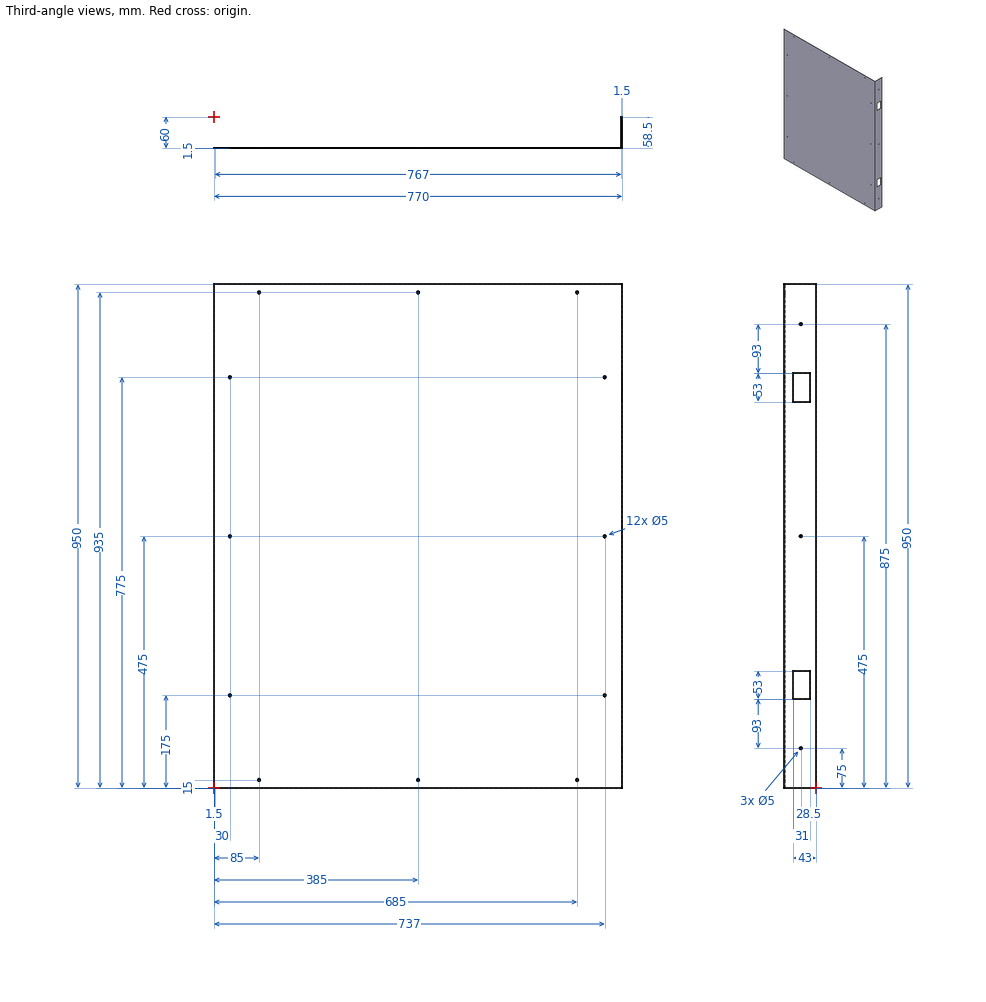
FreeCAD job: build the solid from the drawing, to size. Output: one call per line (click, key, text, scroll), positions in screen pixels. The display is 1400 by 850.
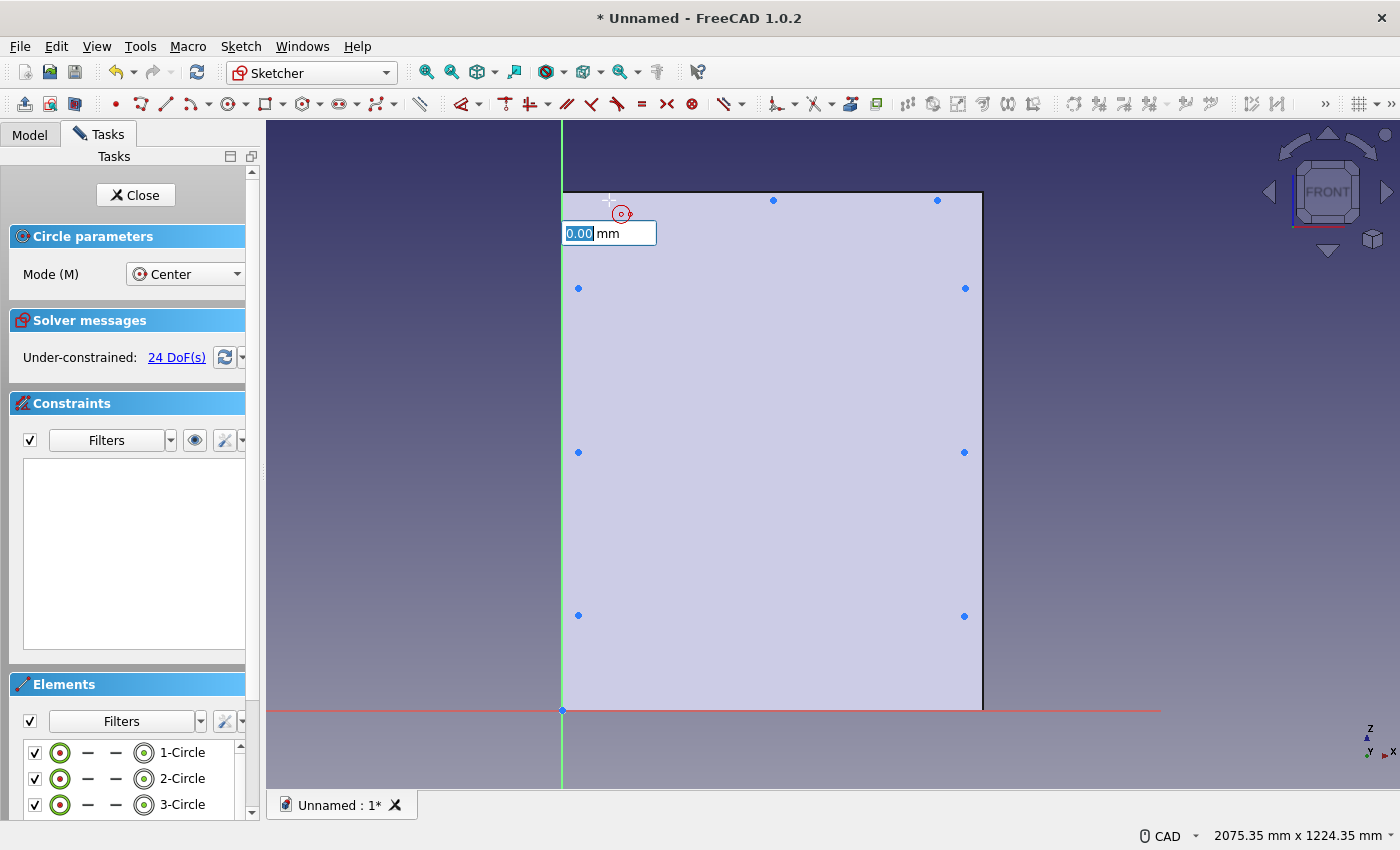
scroll(610, 199, up, 13)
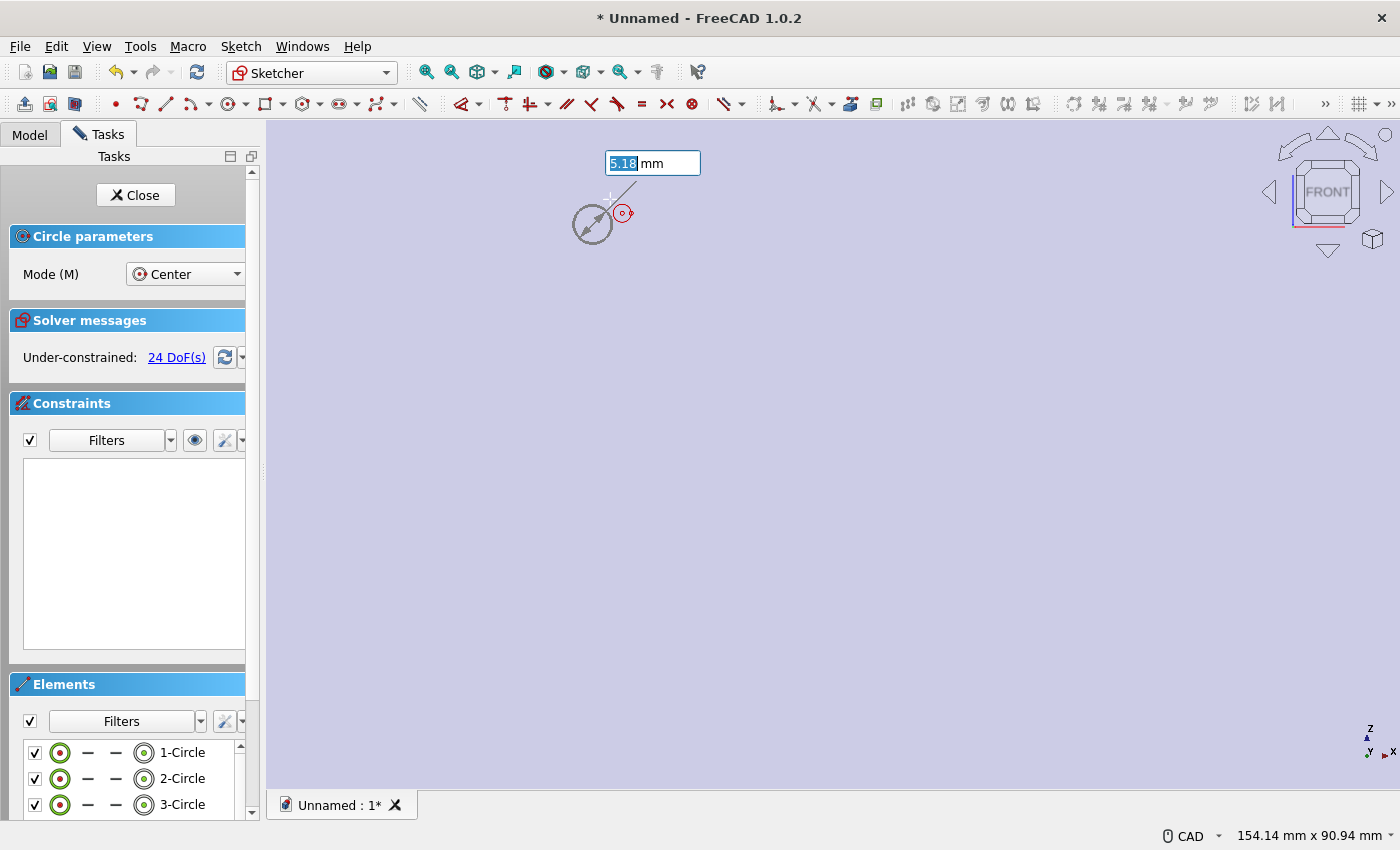
click(604, 196)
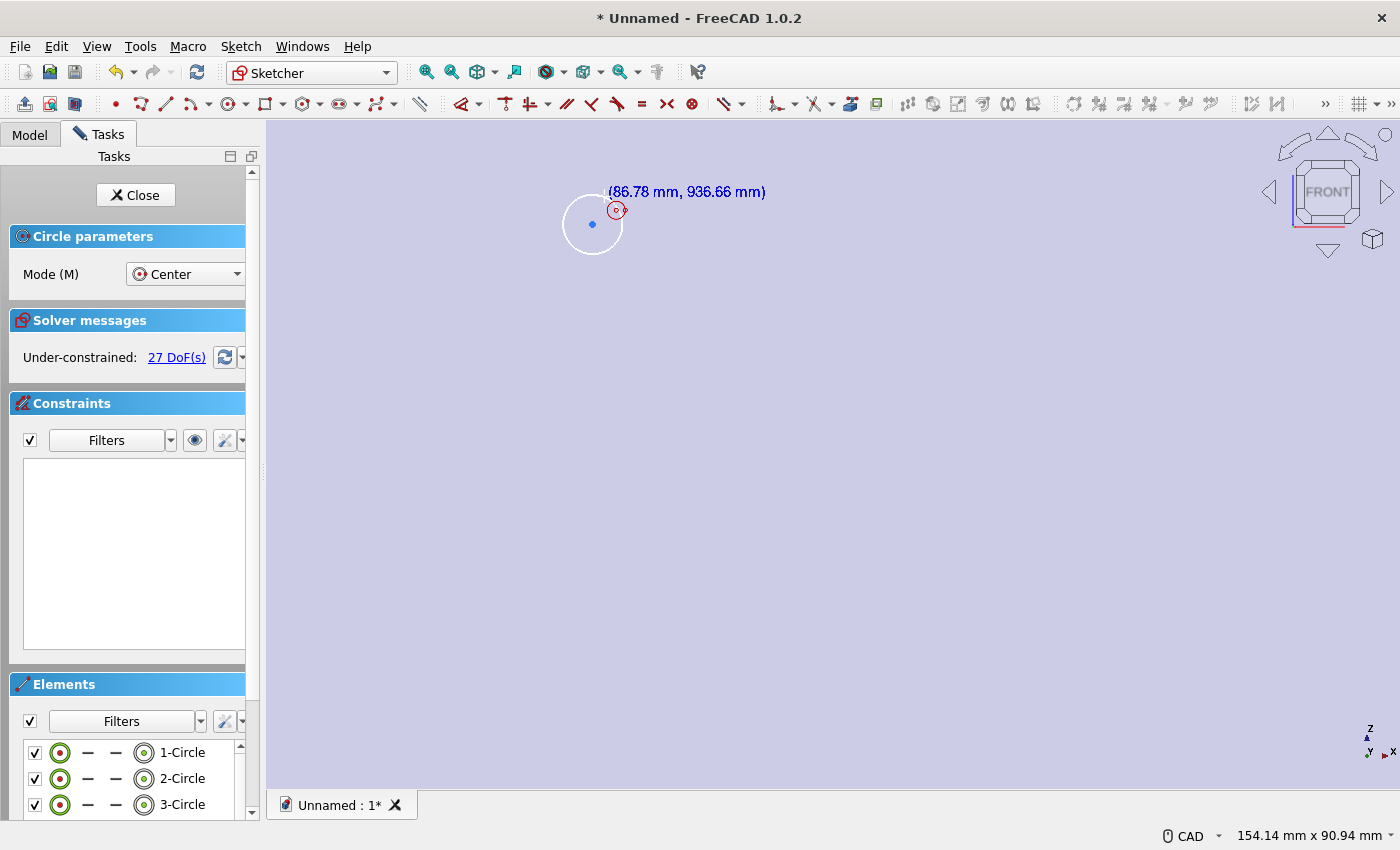
scroll(640, 248, down, 14)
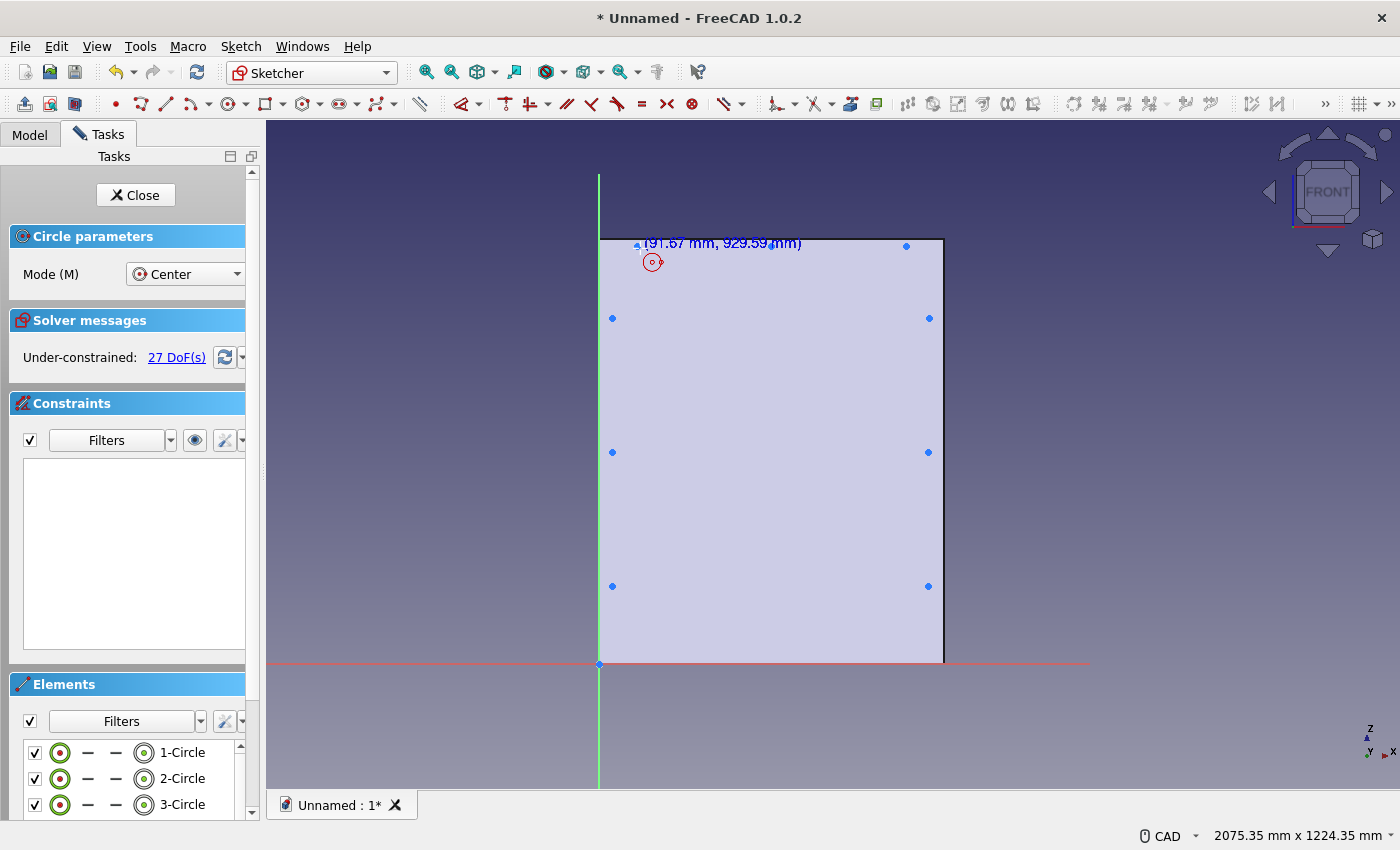
scroll(637, 657, up, 16)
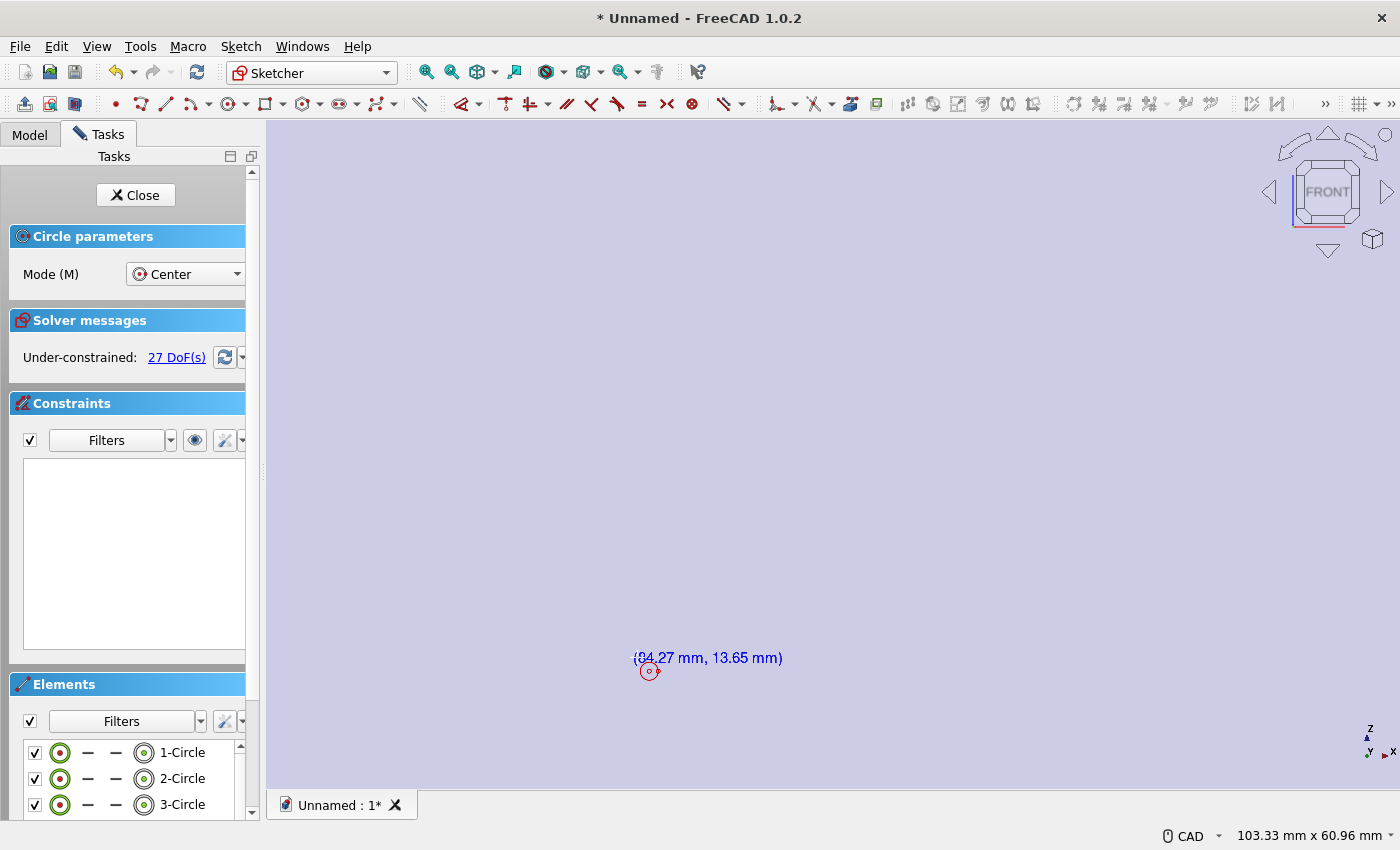
scroll(607, 705, down, 15)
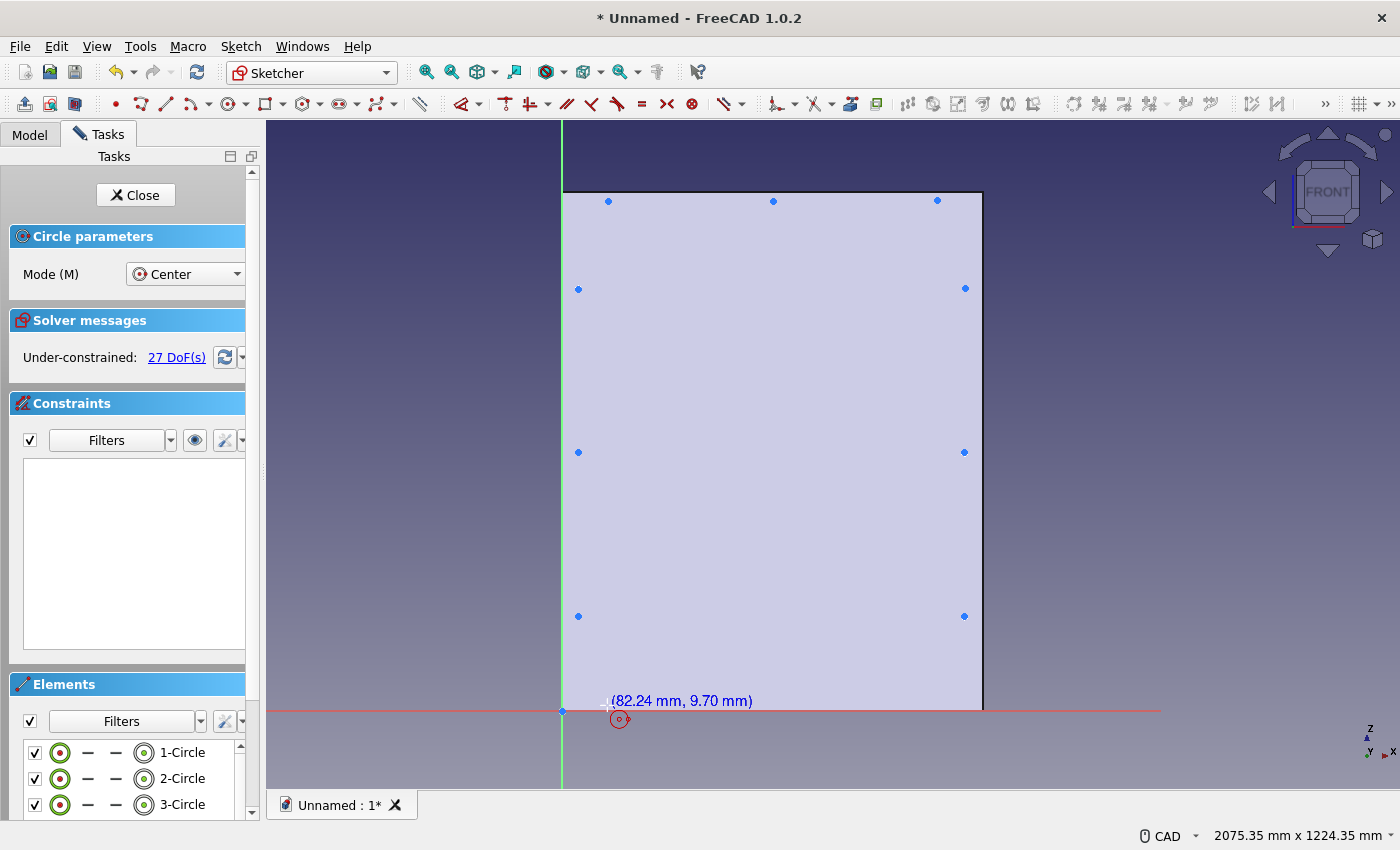
scroll(609, 703, up, 4)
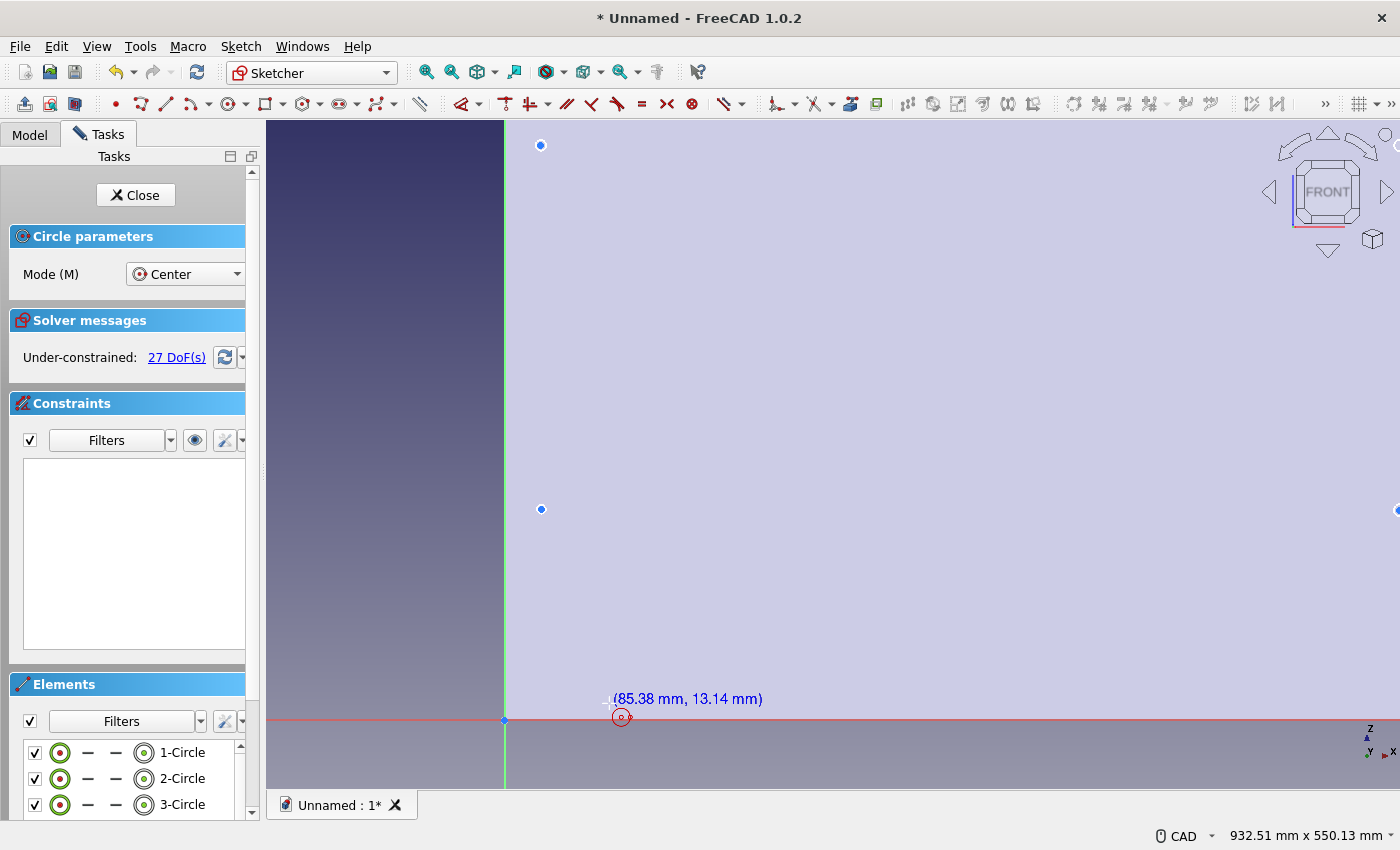
click(608, 702)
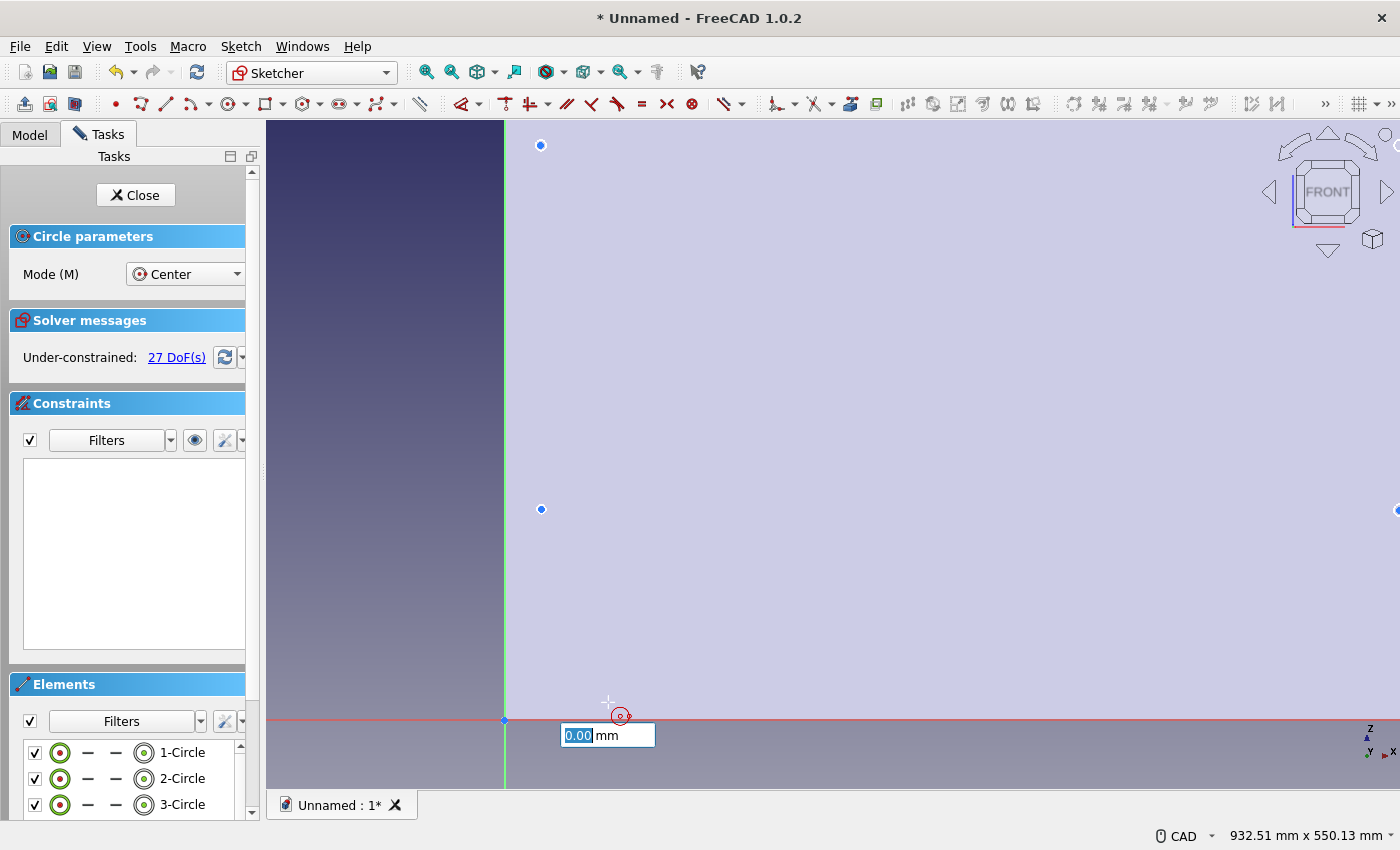
scroll(610, 700, up, 9)